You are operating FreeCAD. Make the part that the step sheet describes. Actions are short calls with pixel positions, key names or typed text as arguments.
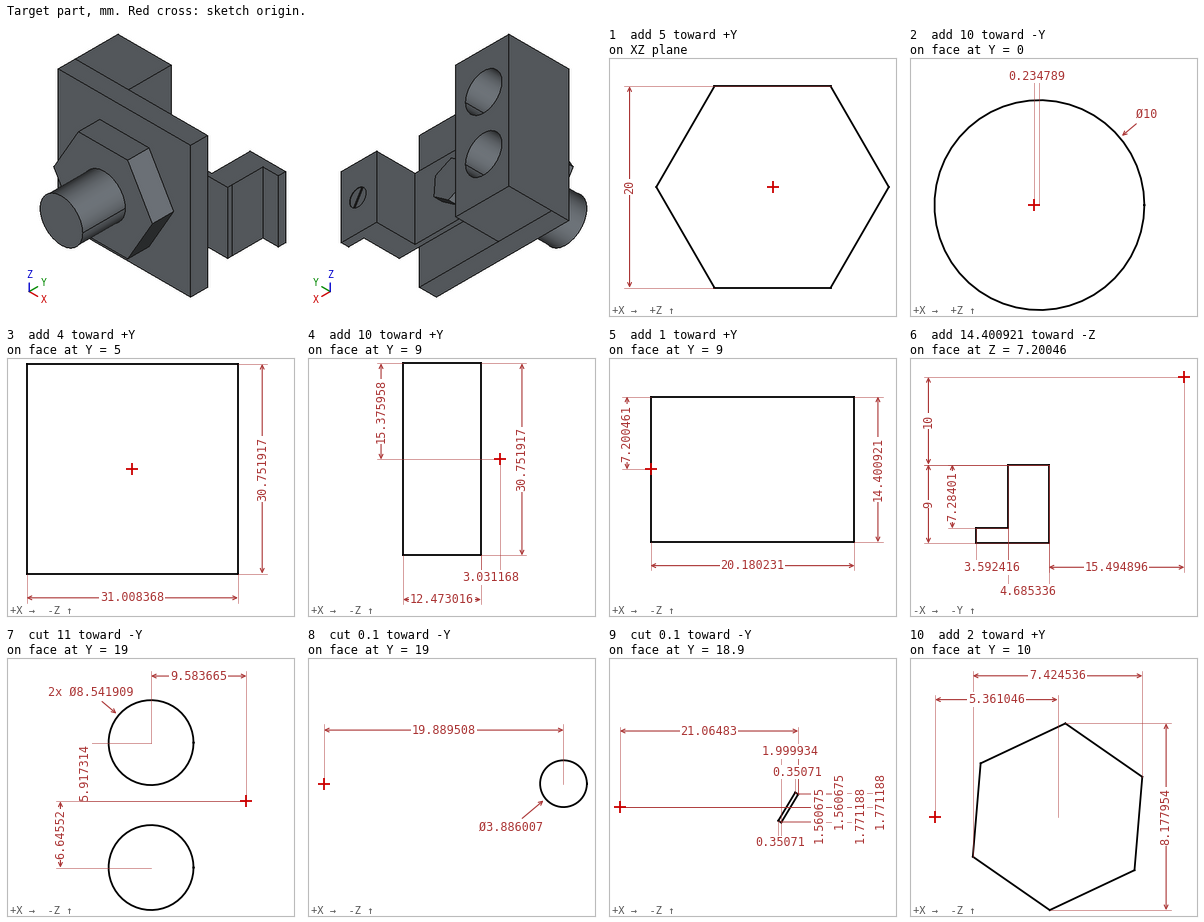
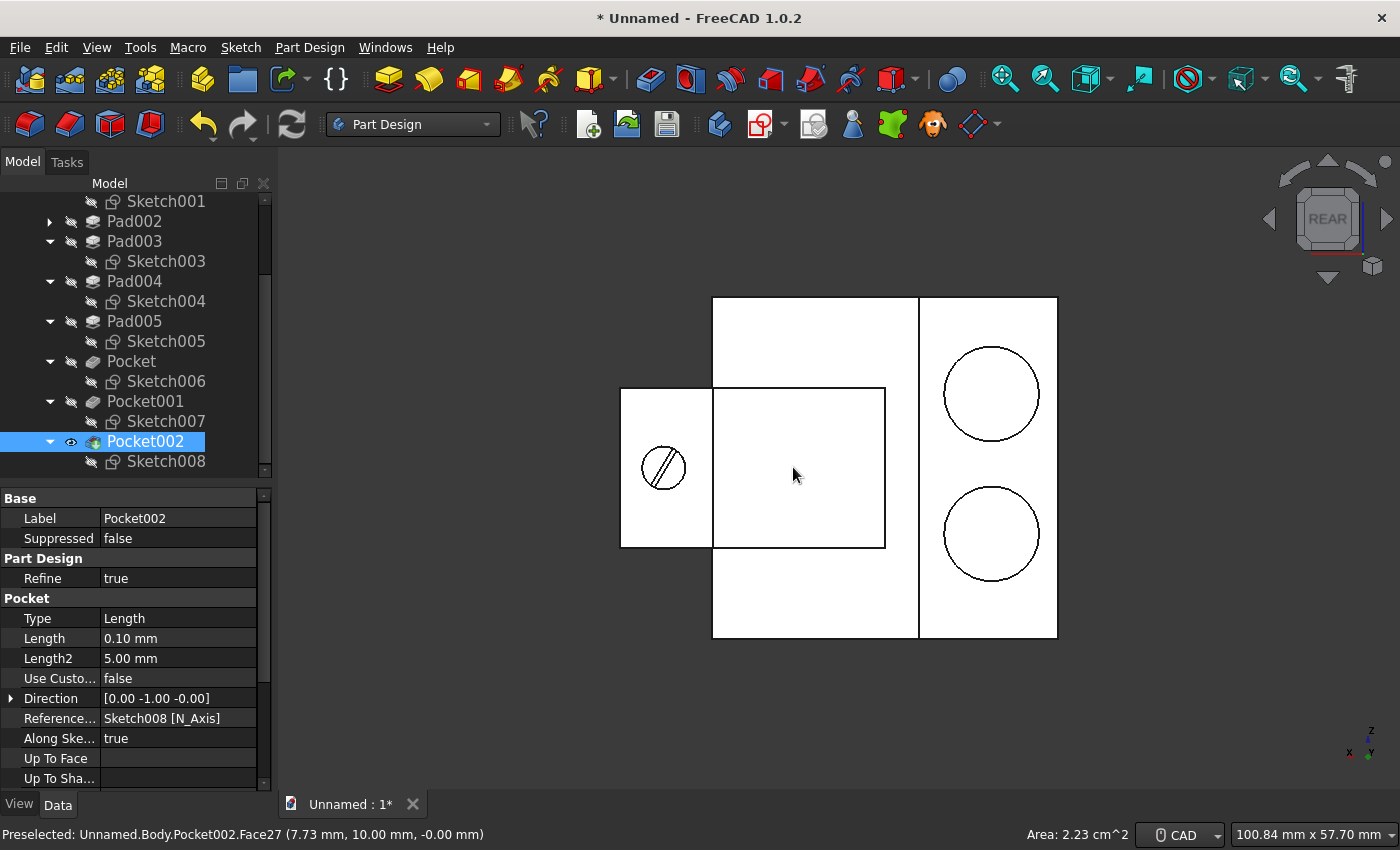
click(760, 124)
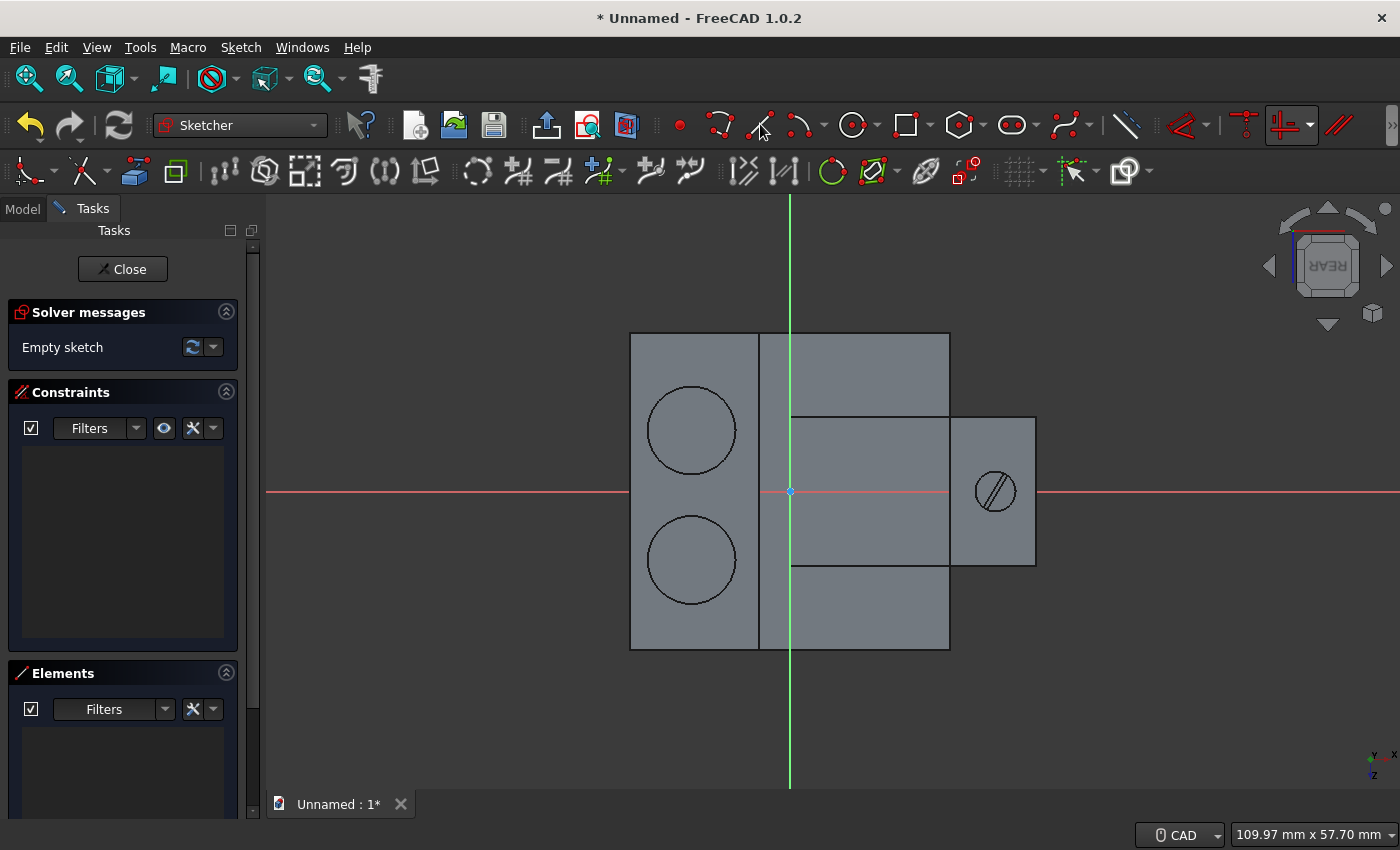
scroll(856, 491, up, 8)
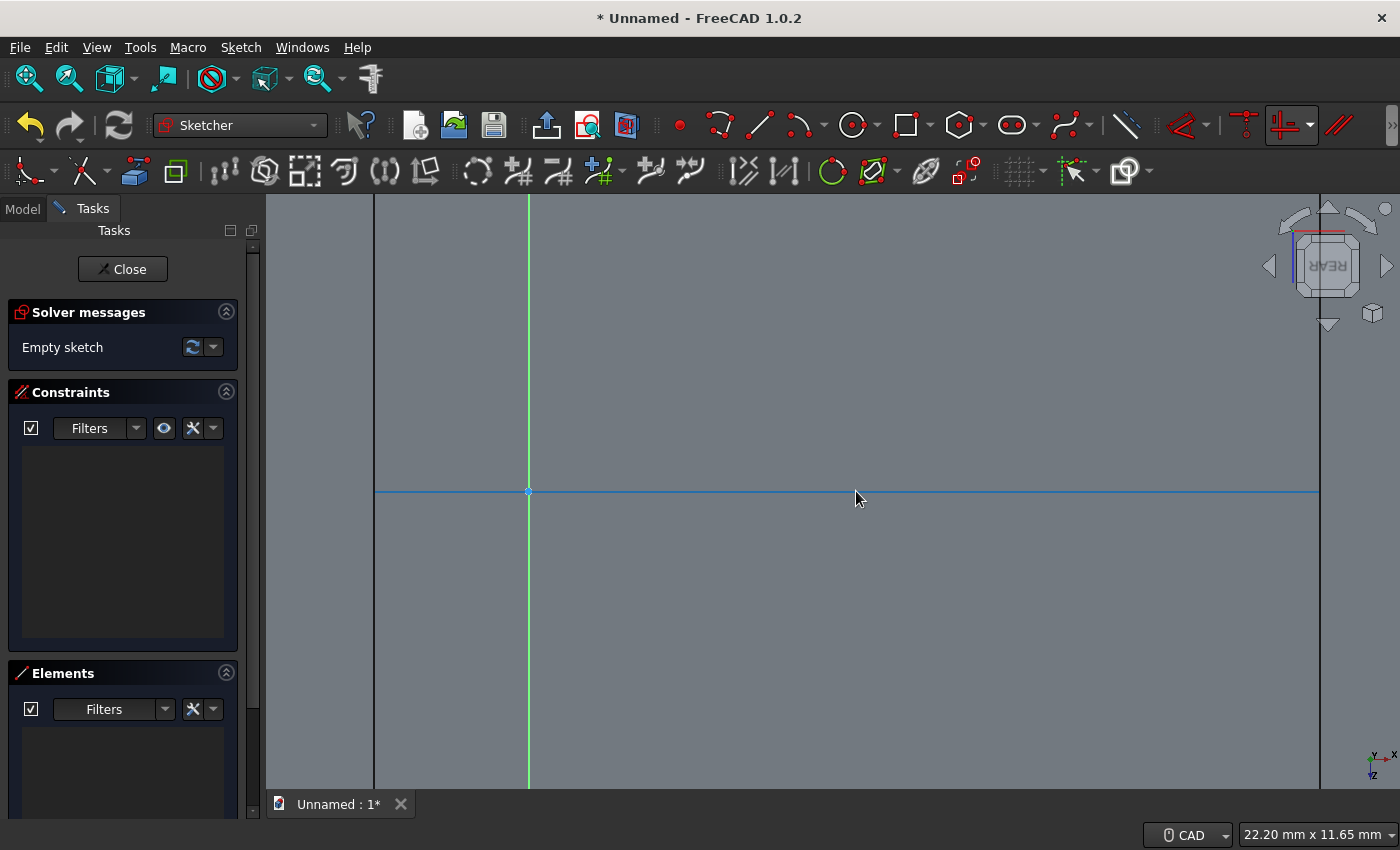
click(960, 126)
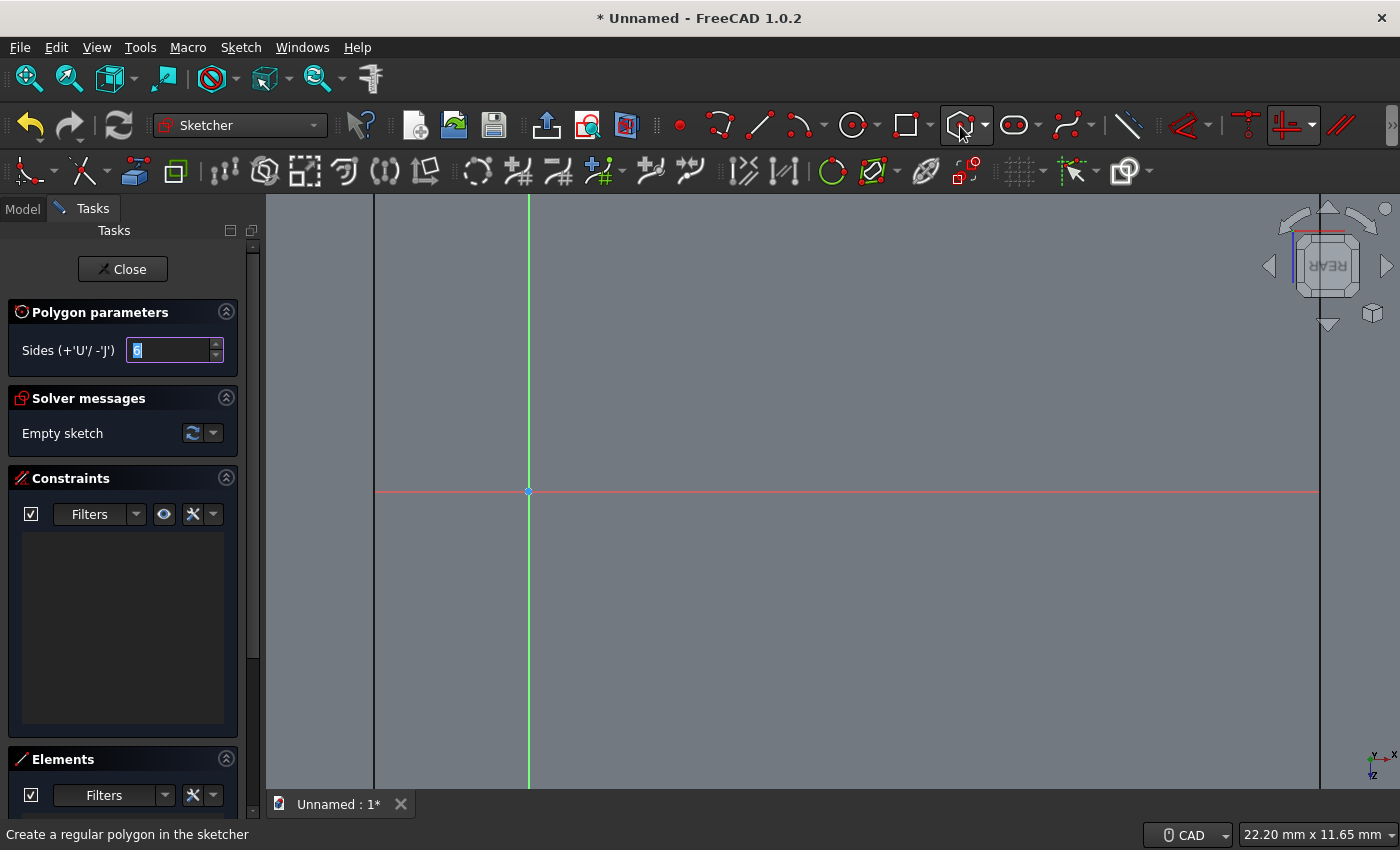
click(803, 491)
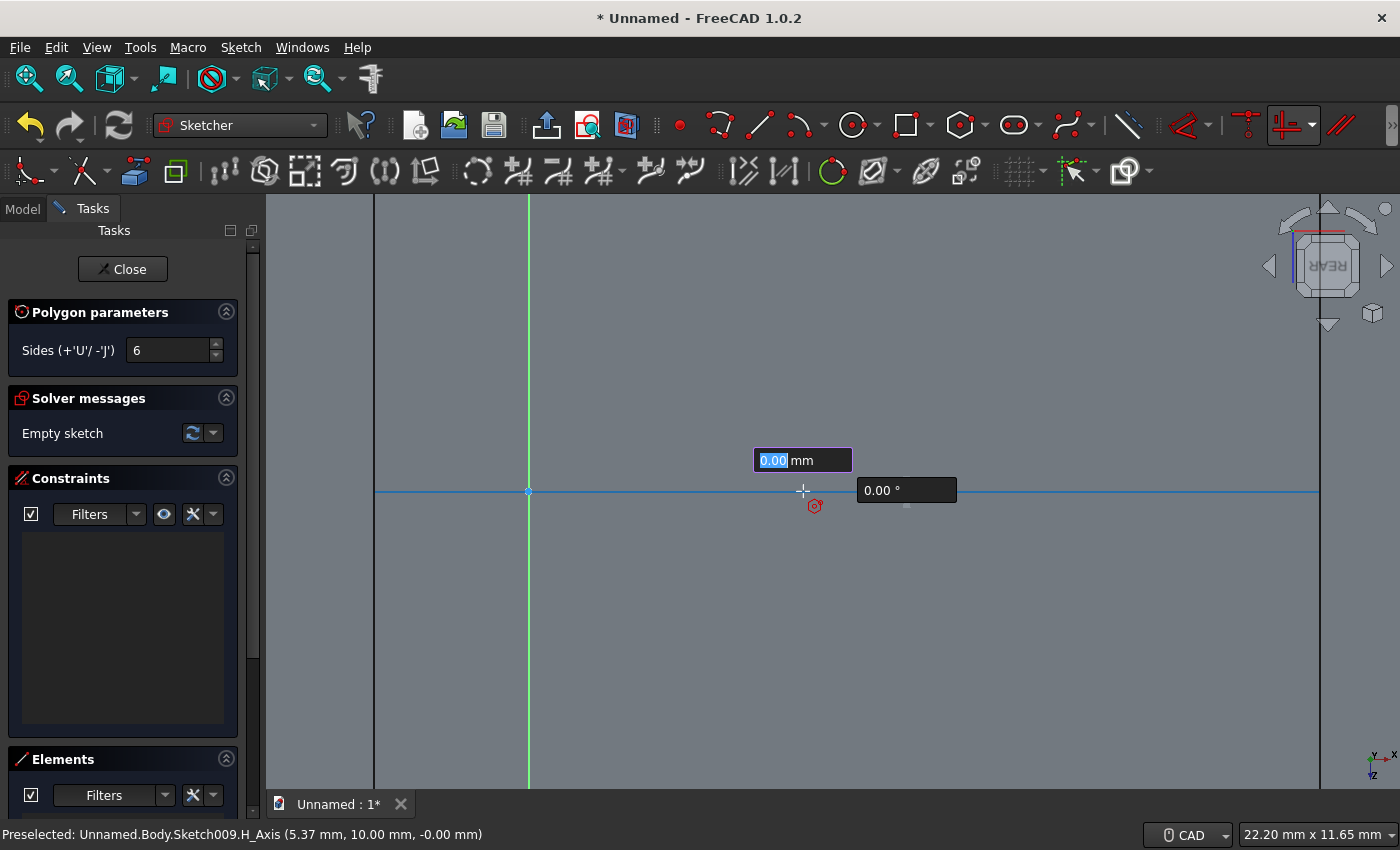
click(820, 283)
right_click(820, 283)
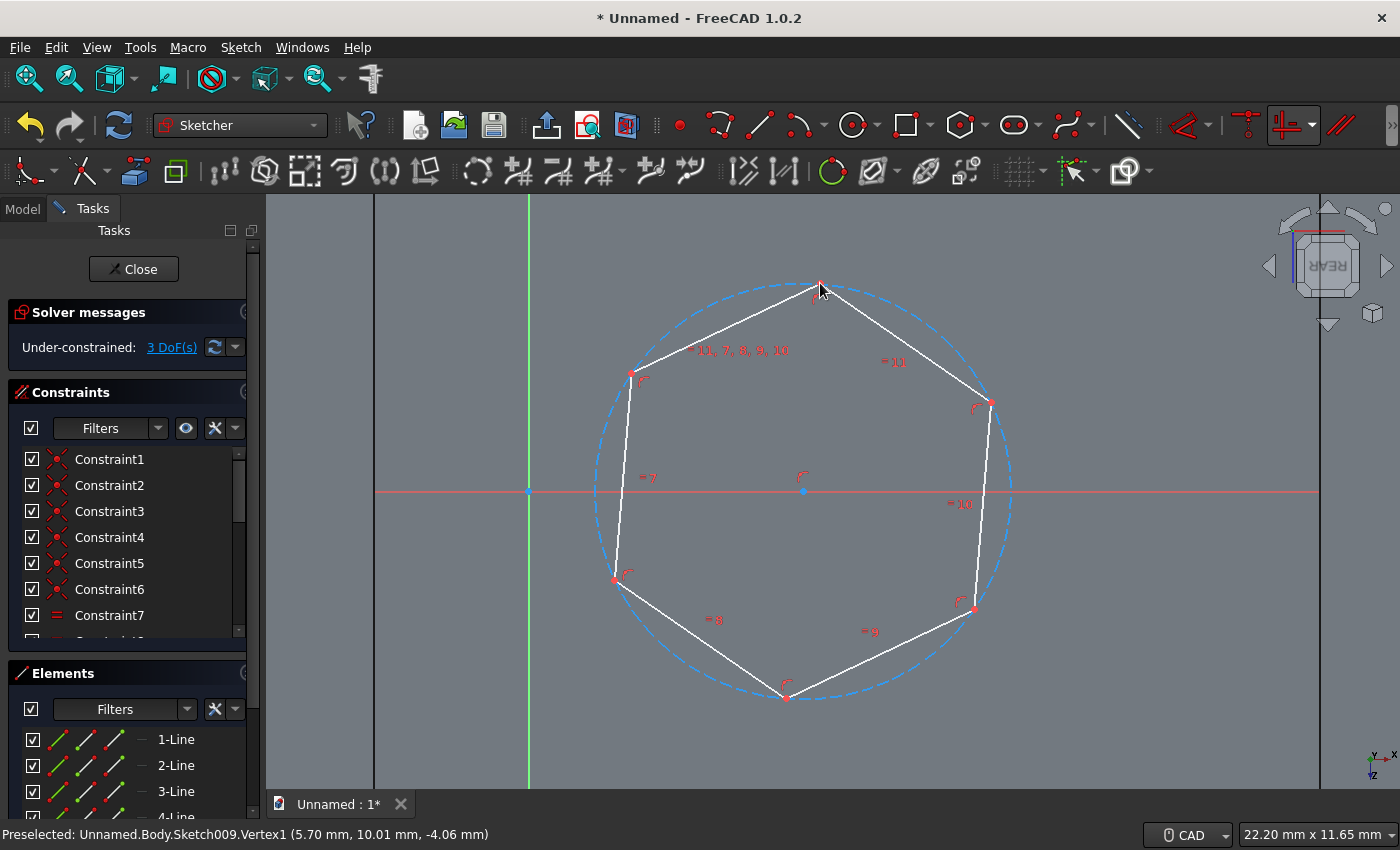
click(1184, 126)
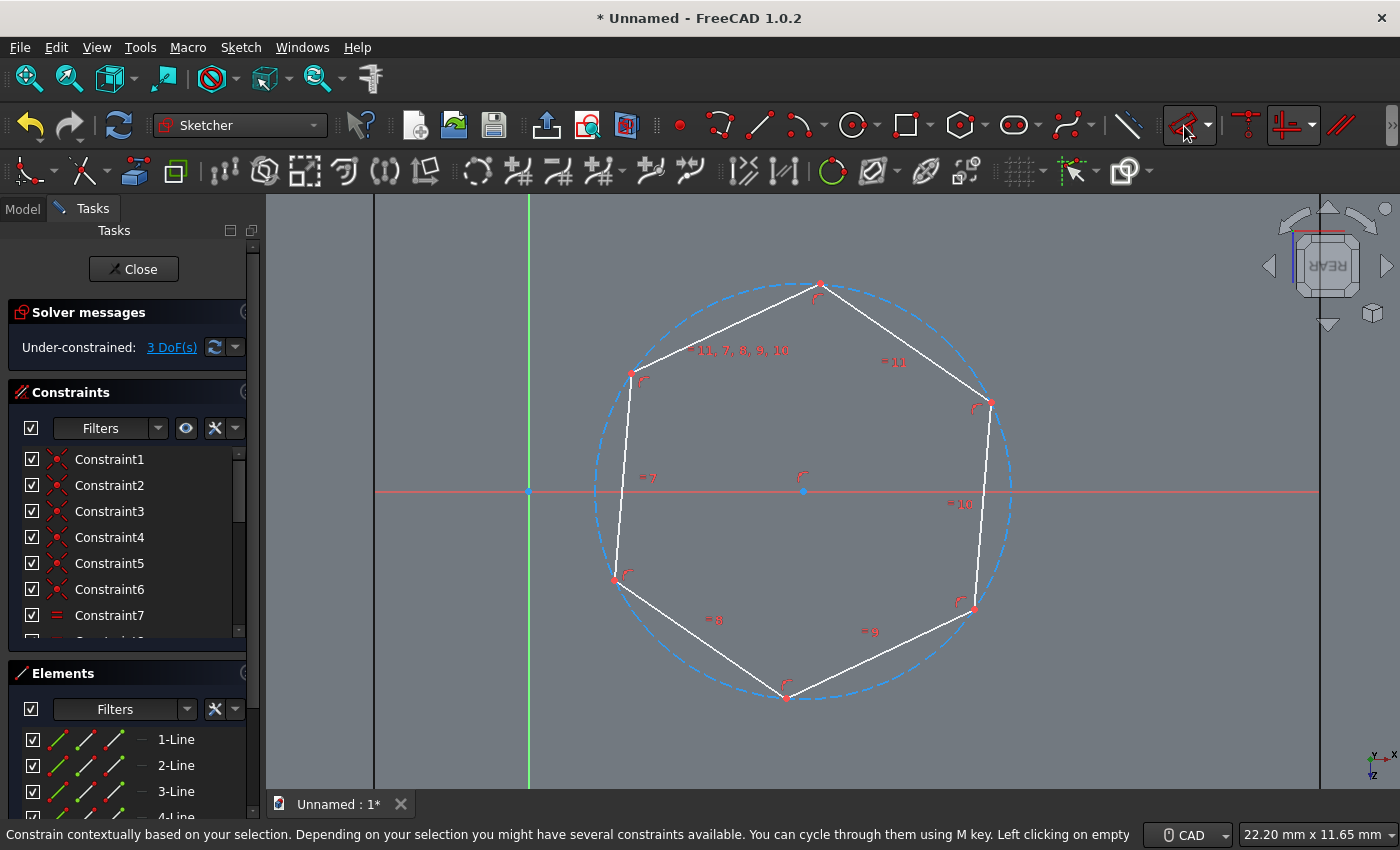
click(615, 581)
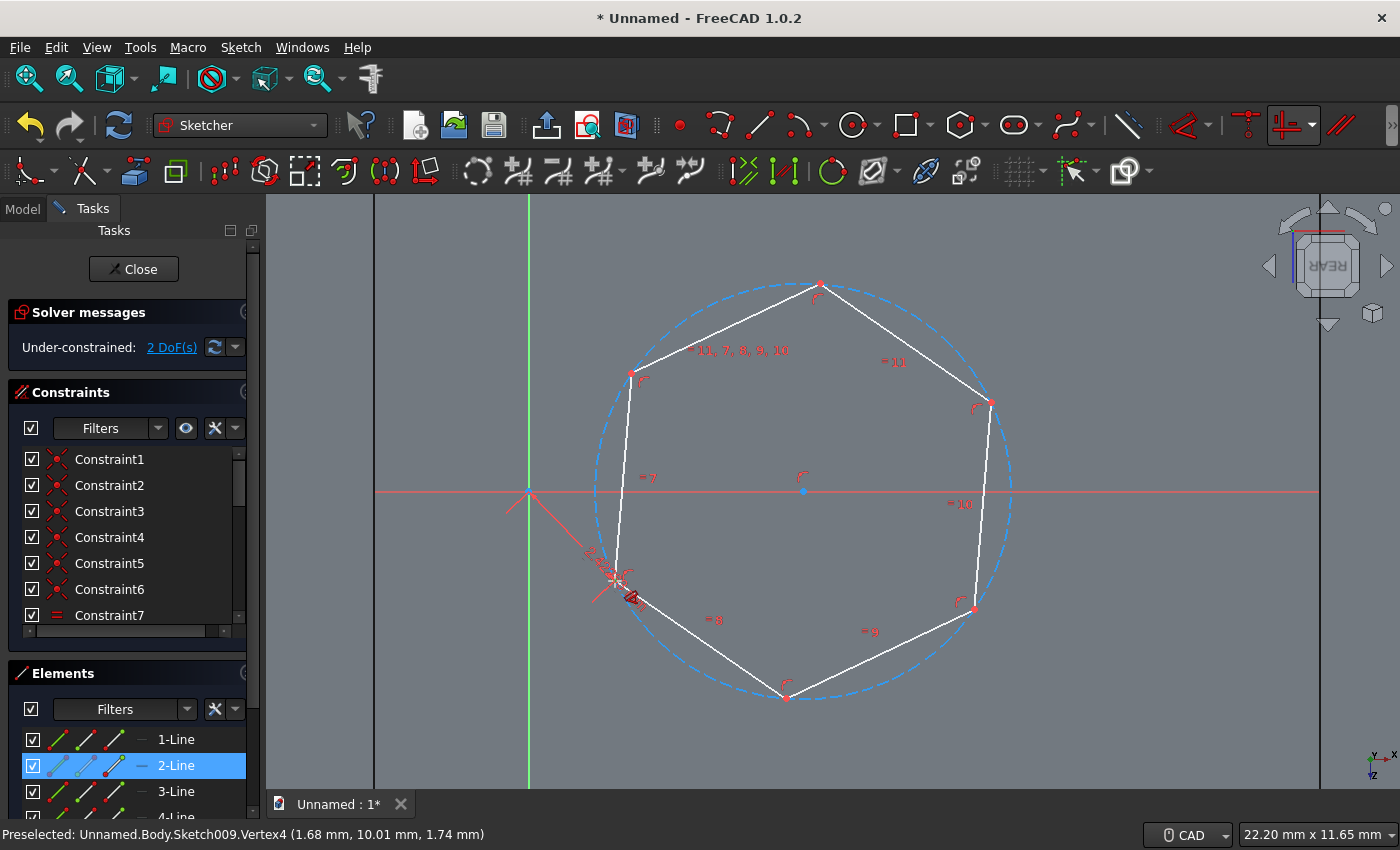
click(991, 402)
click(803, 615)